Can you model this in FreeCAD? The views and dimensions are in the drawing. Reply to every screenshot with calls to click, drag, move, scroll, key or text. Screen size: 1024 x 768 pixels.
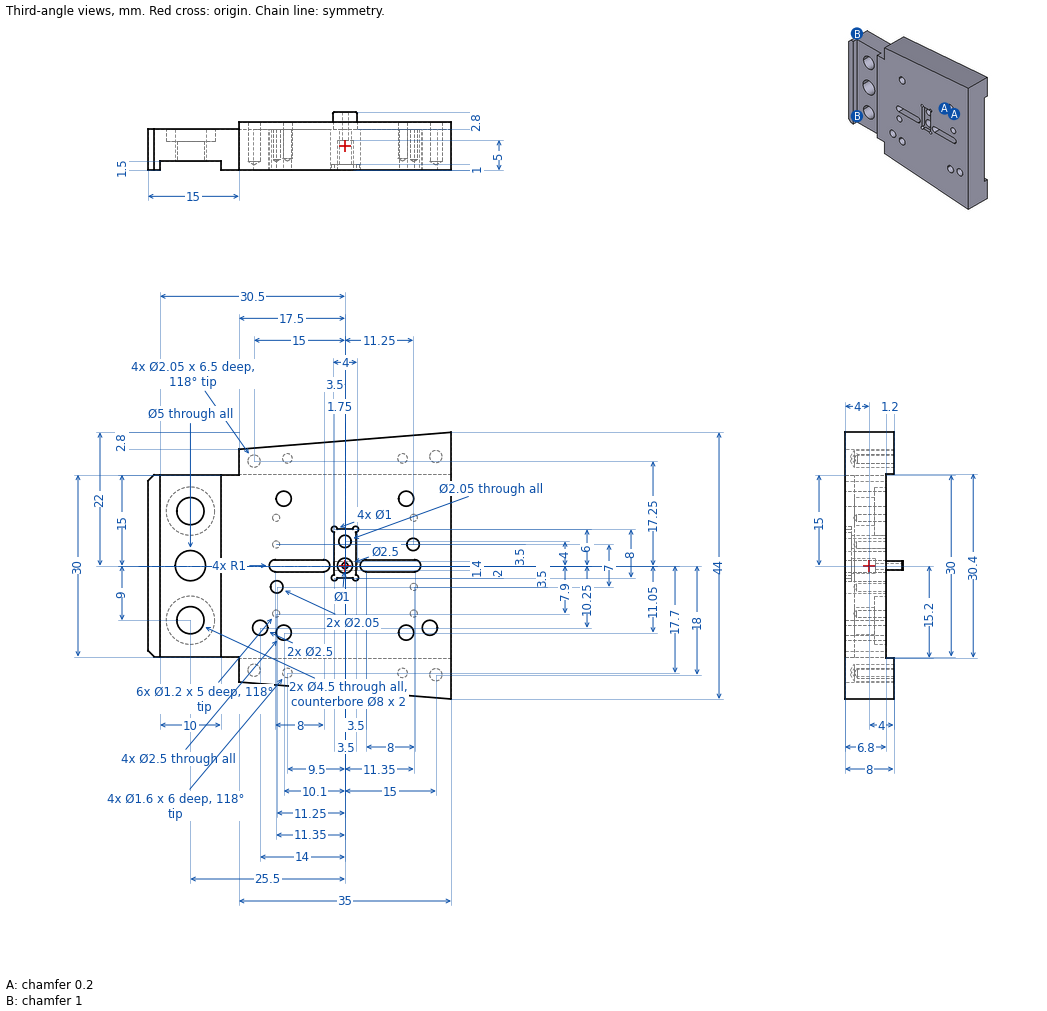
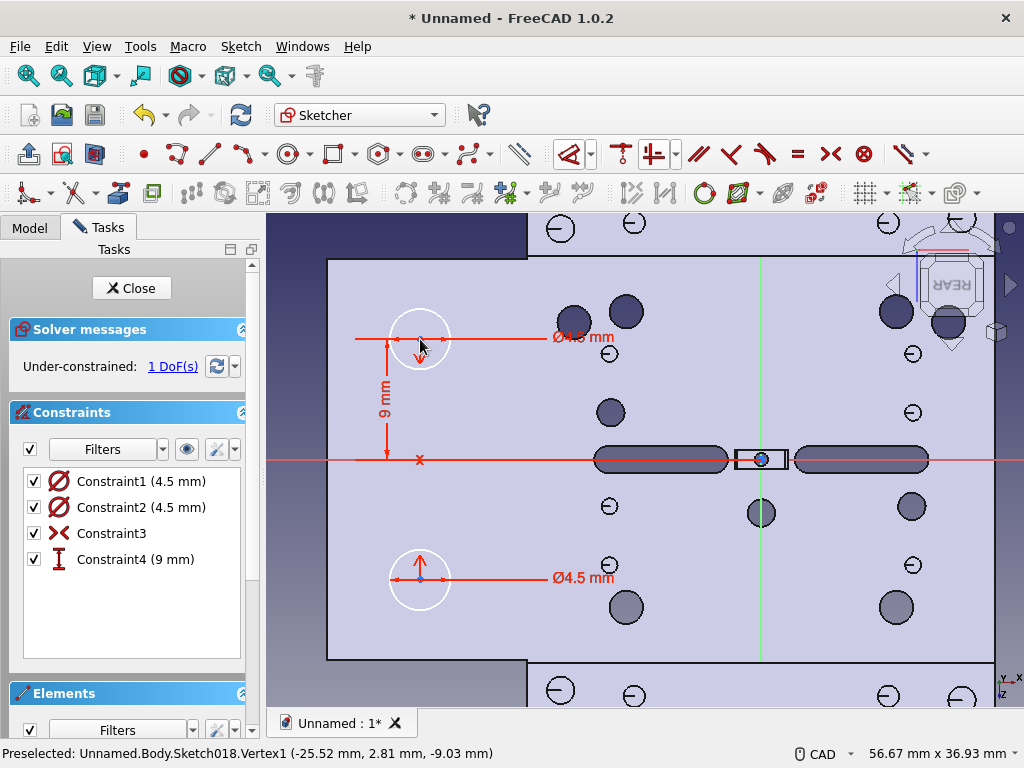
click(420, 339)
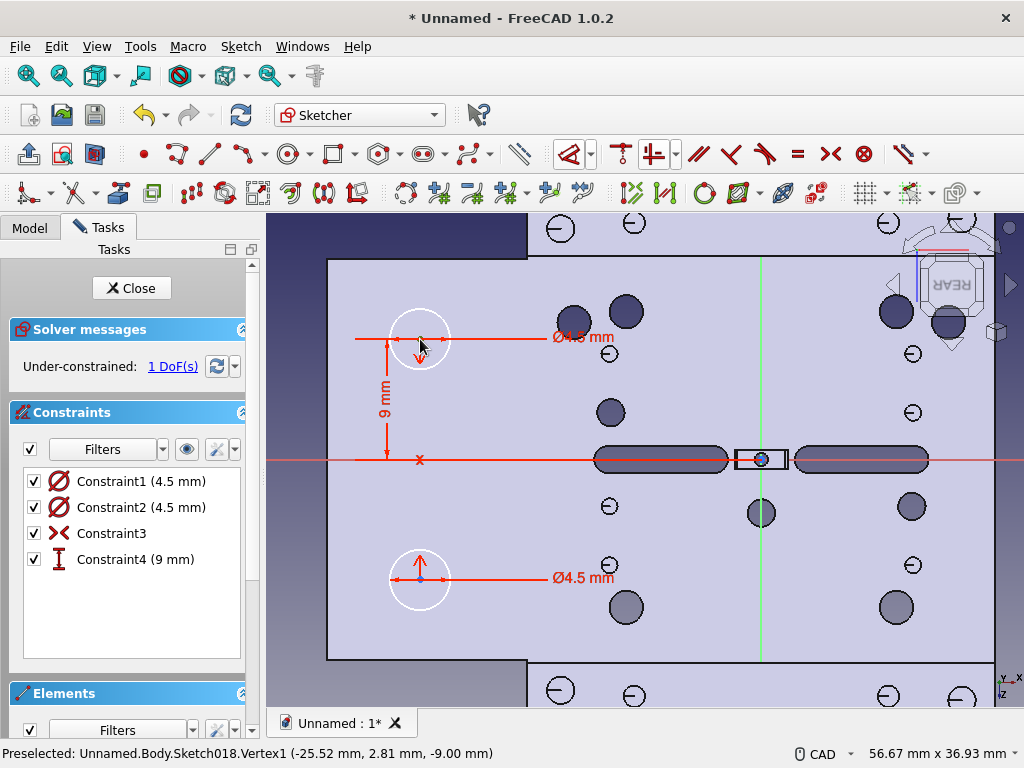
click(590, 154)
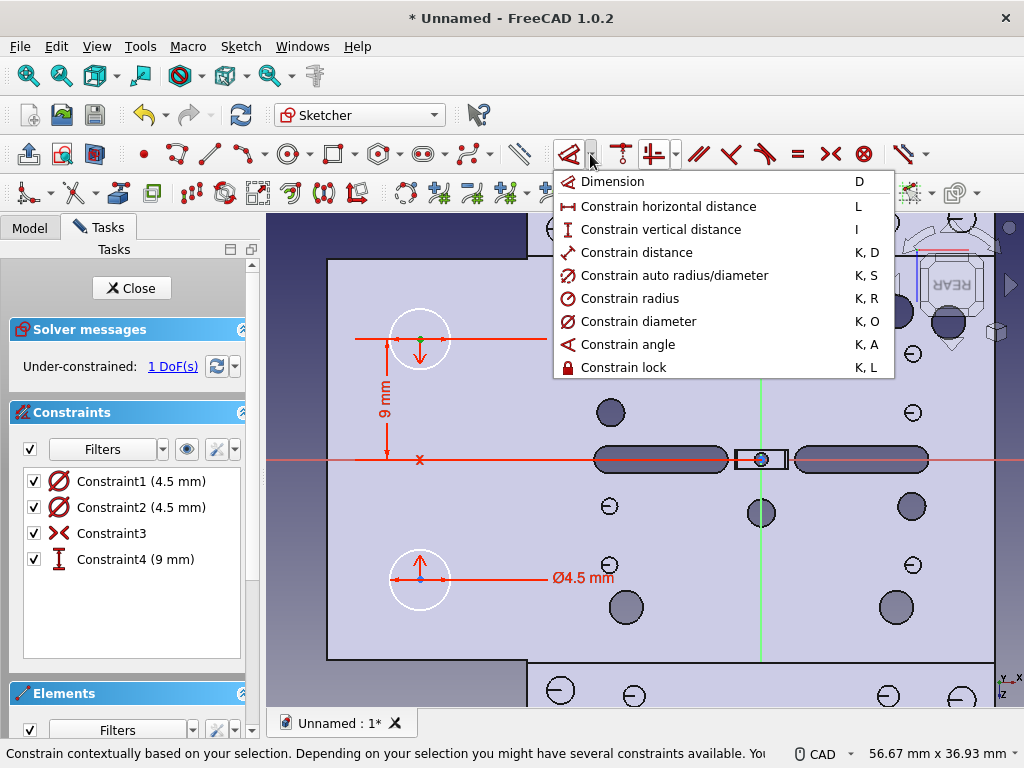
click(724, 206)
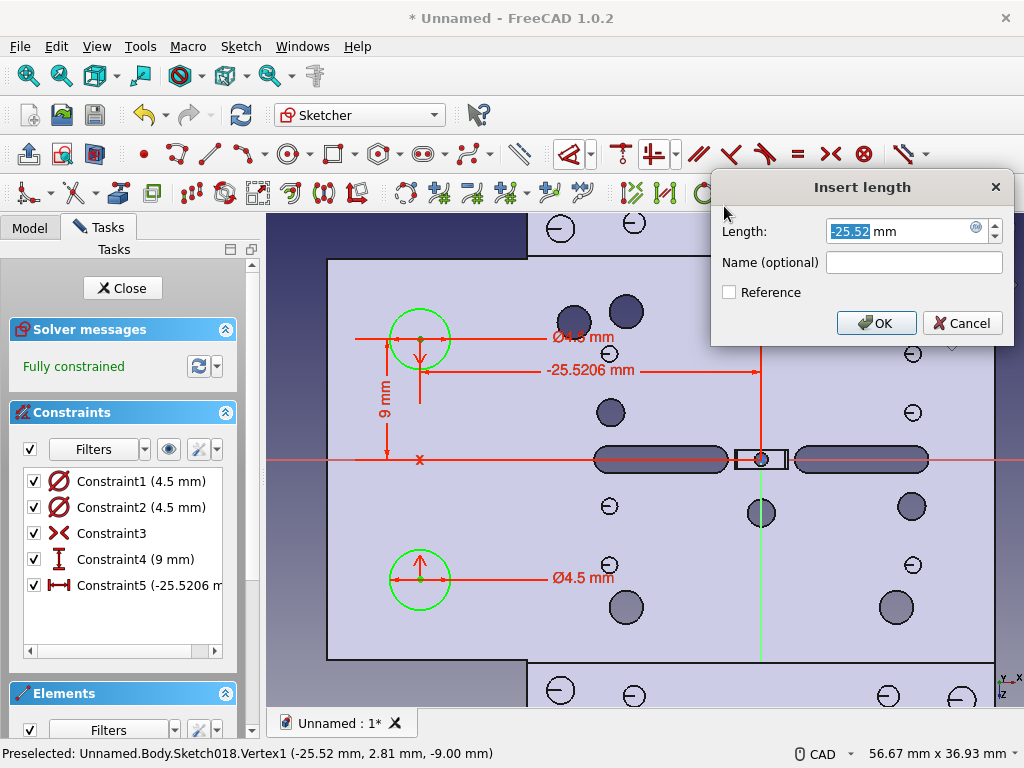
text(-25.5)
key(Return)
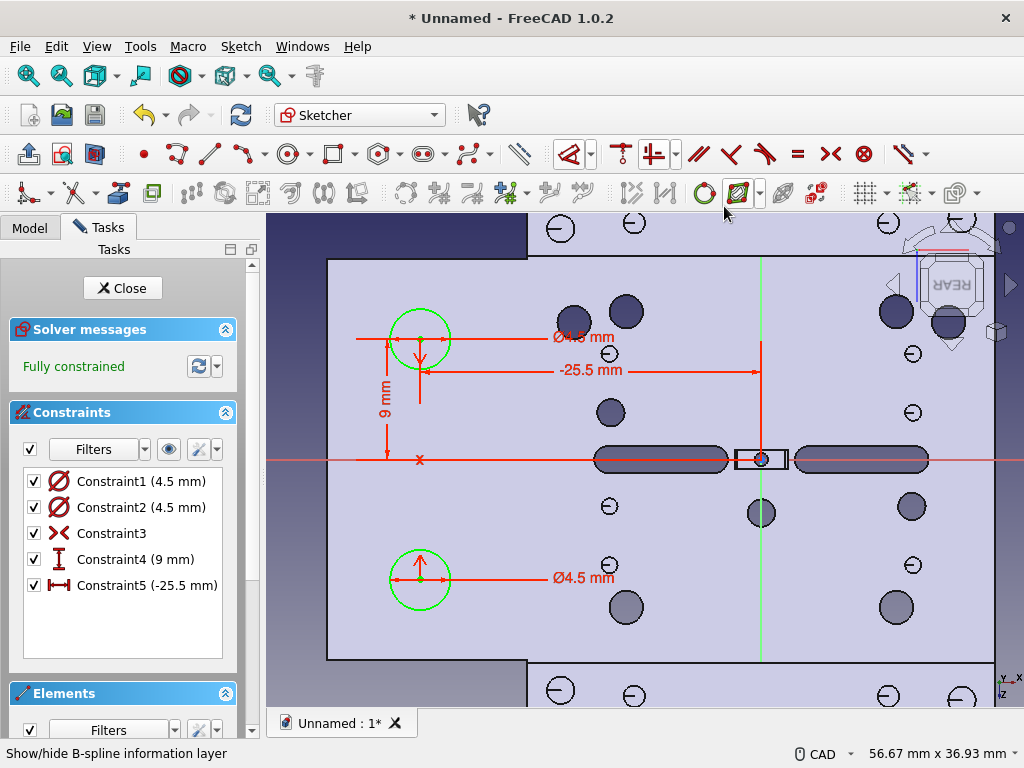
click(123, 288)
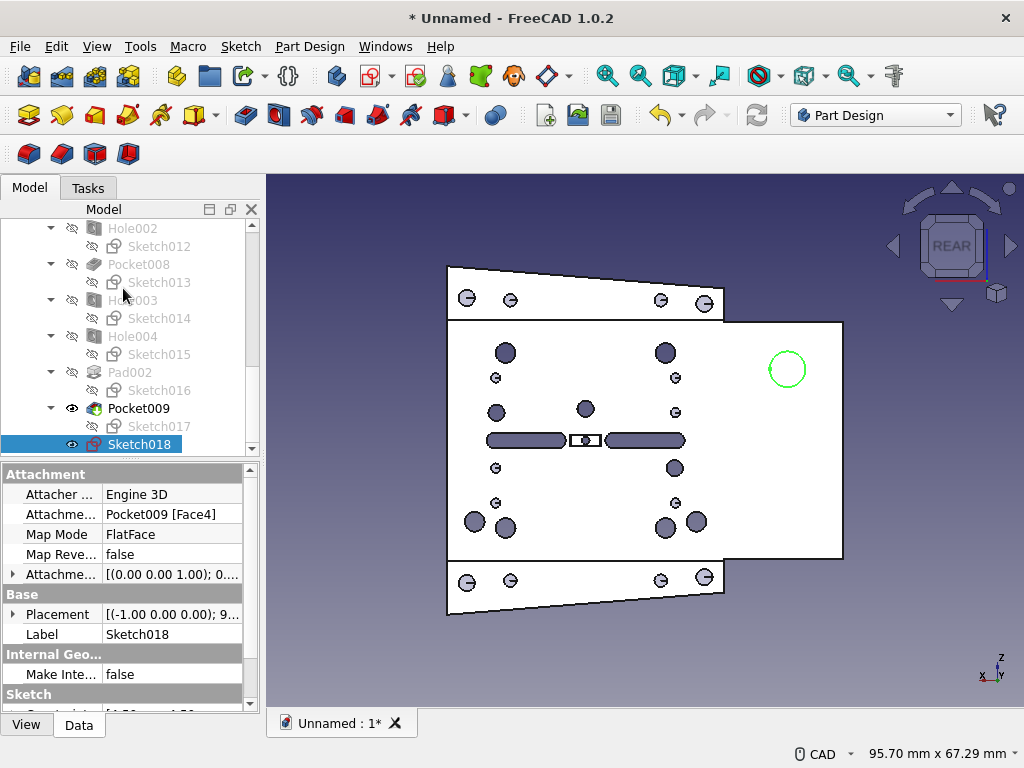
click(279, 116)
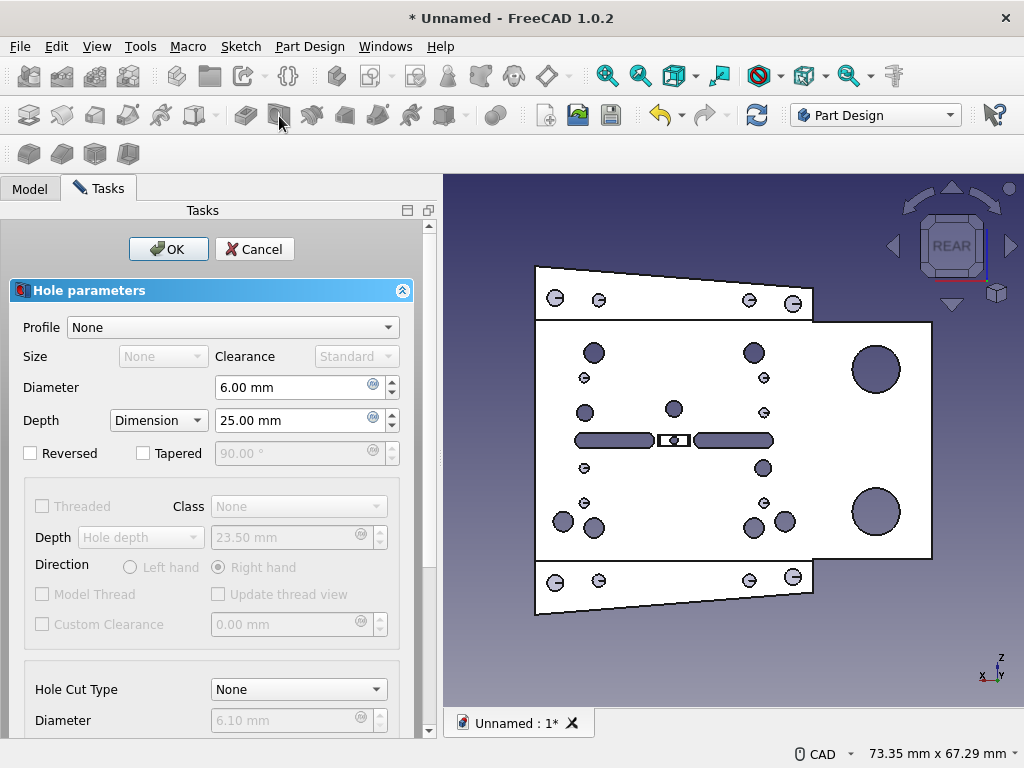
triple_click(300, 388)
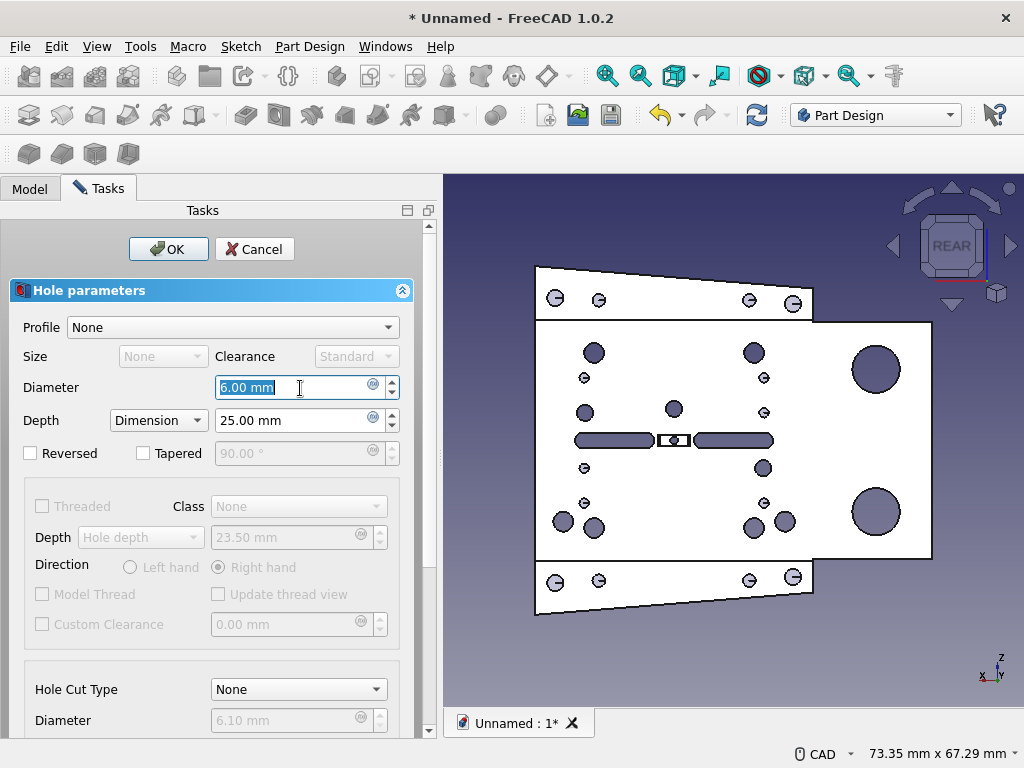
text(4.5)
key(Tab)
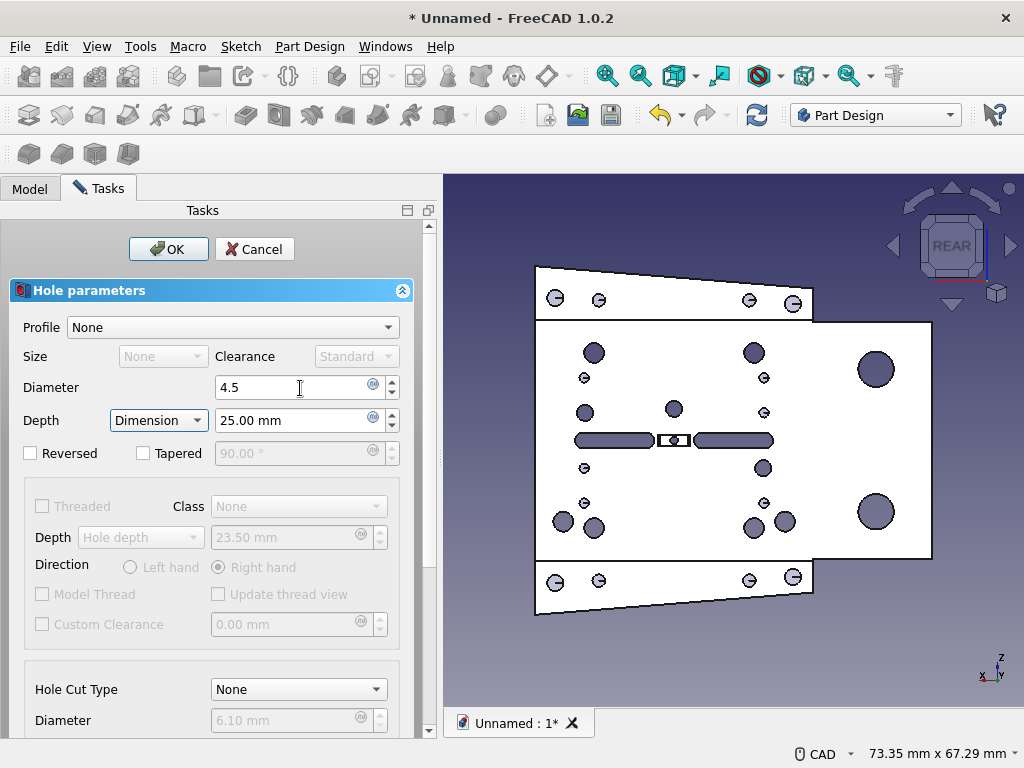
click(160, 420)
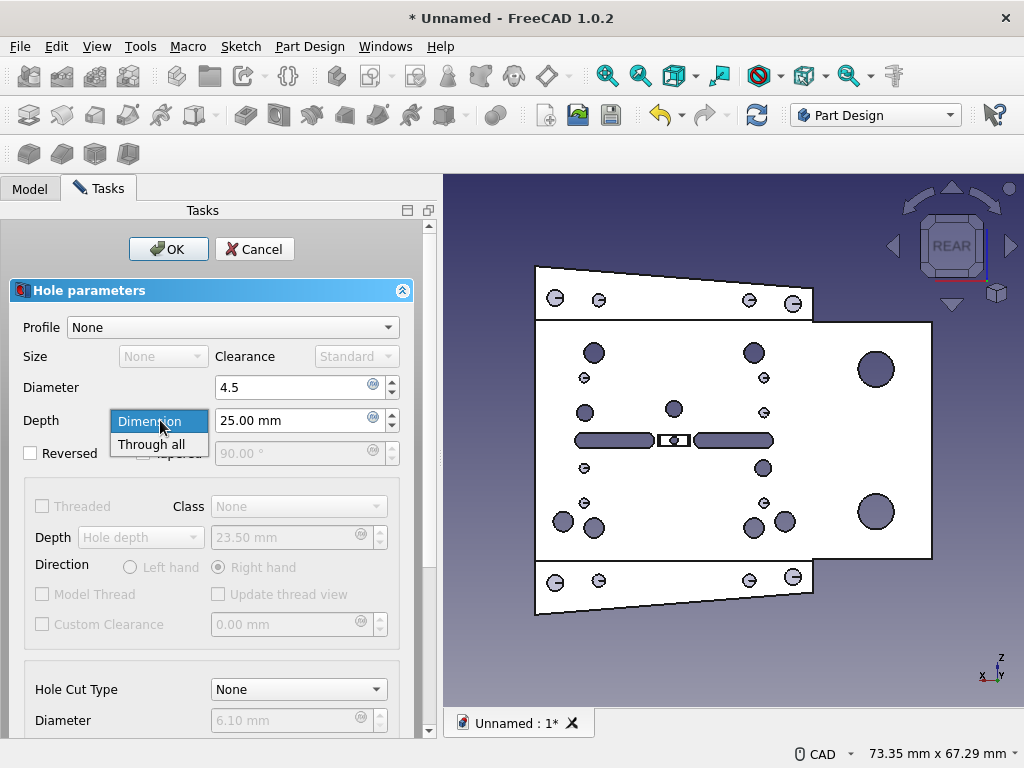
click(158, 444)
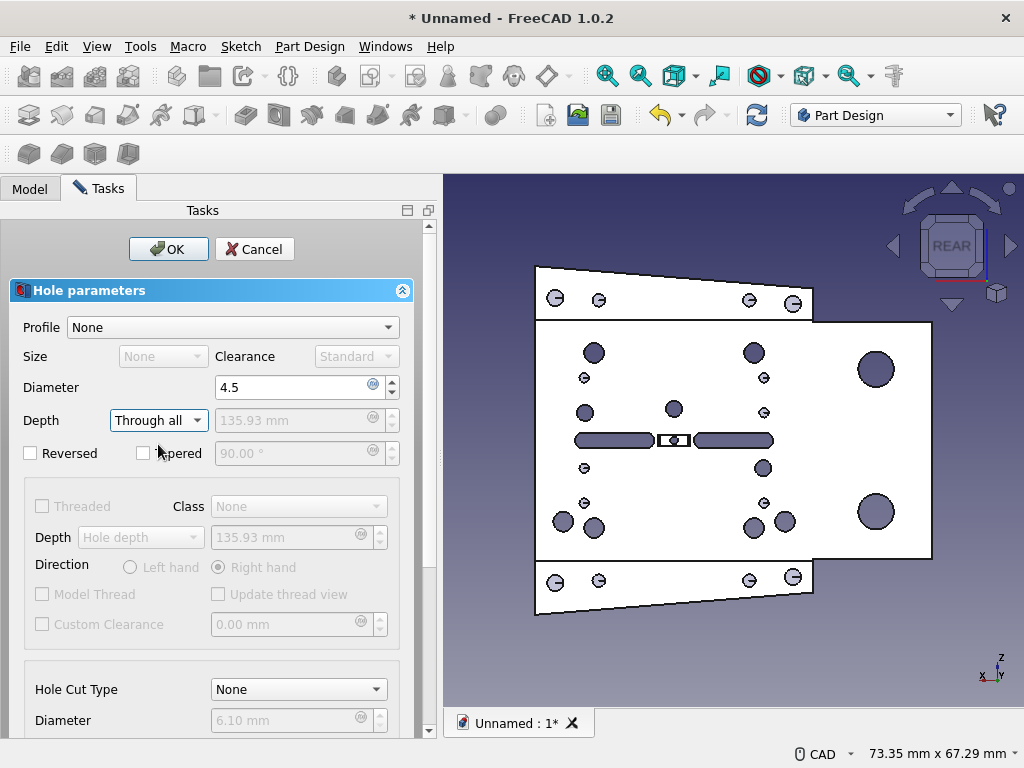
click(300, 690)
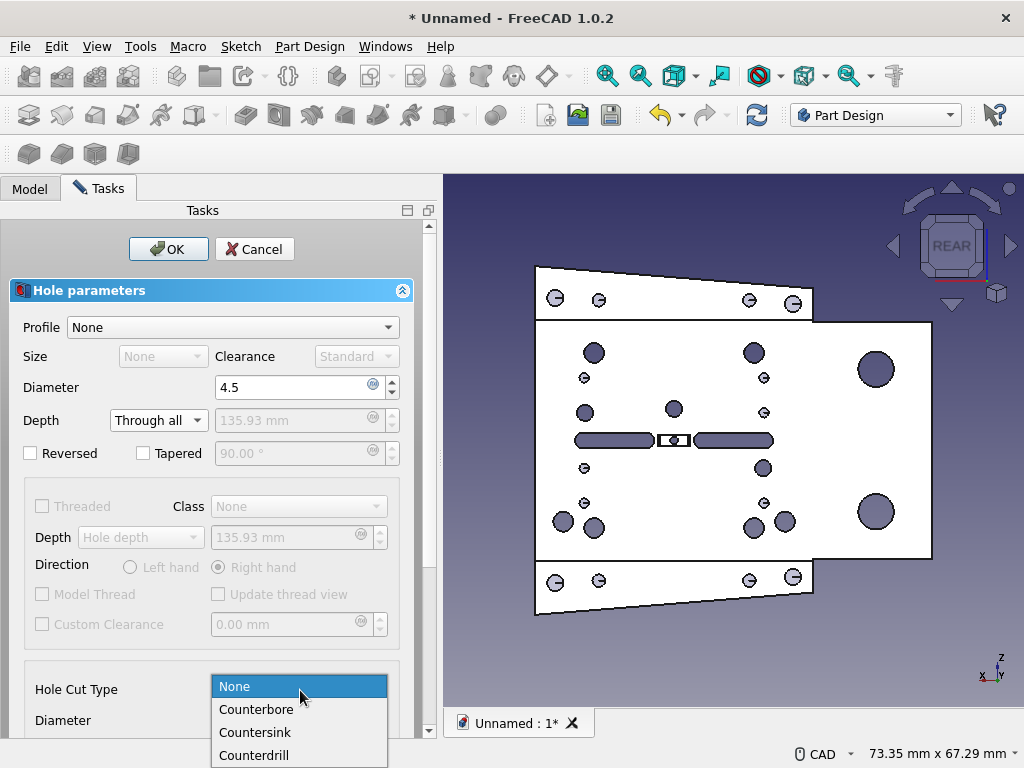
click(298, 710)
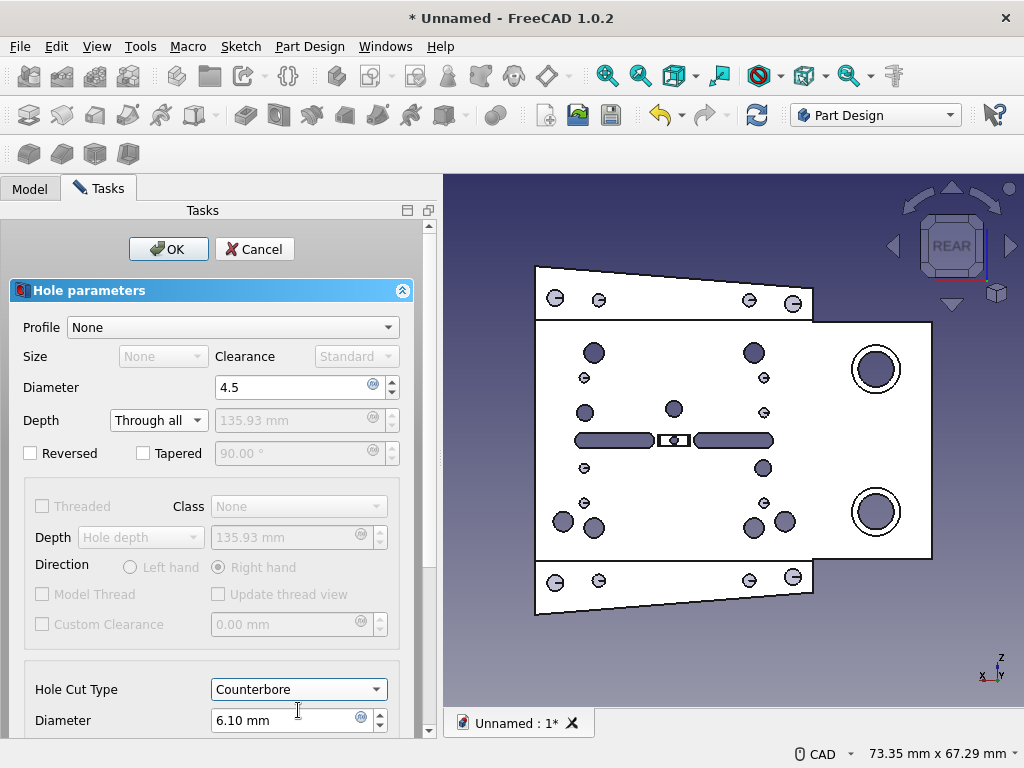
triple_click(292, 720)